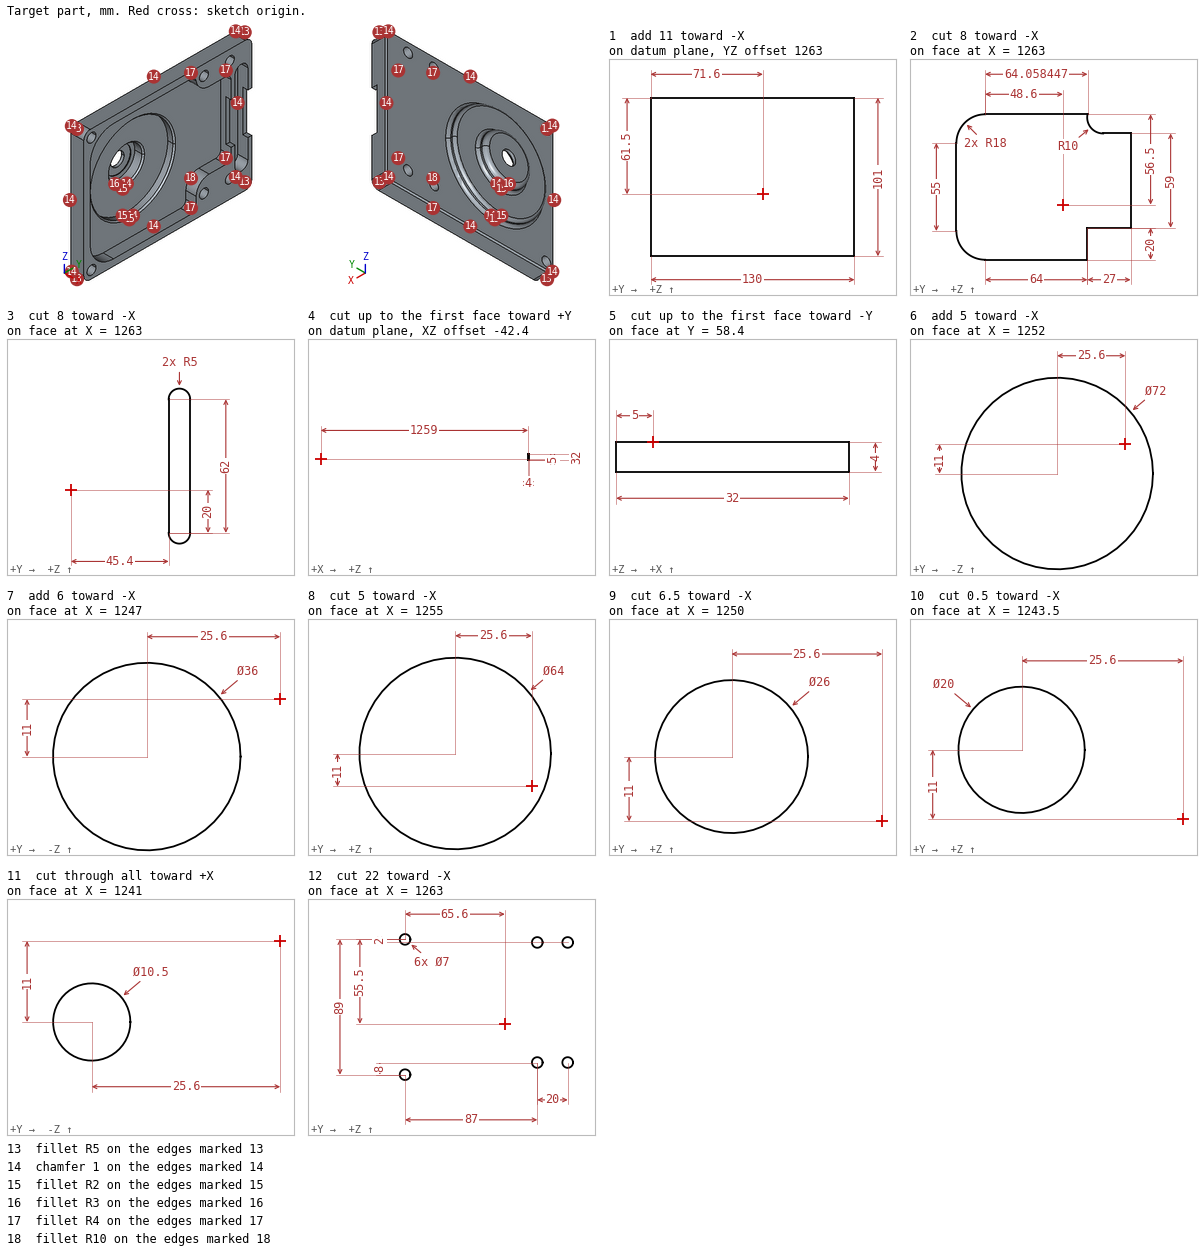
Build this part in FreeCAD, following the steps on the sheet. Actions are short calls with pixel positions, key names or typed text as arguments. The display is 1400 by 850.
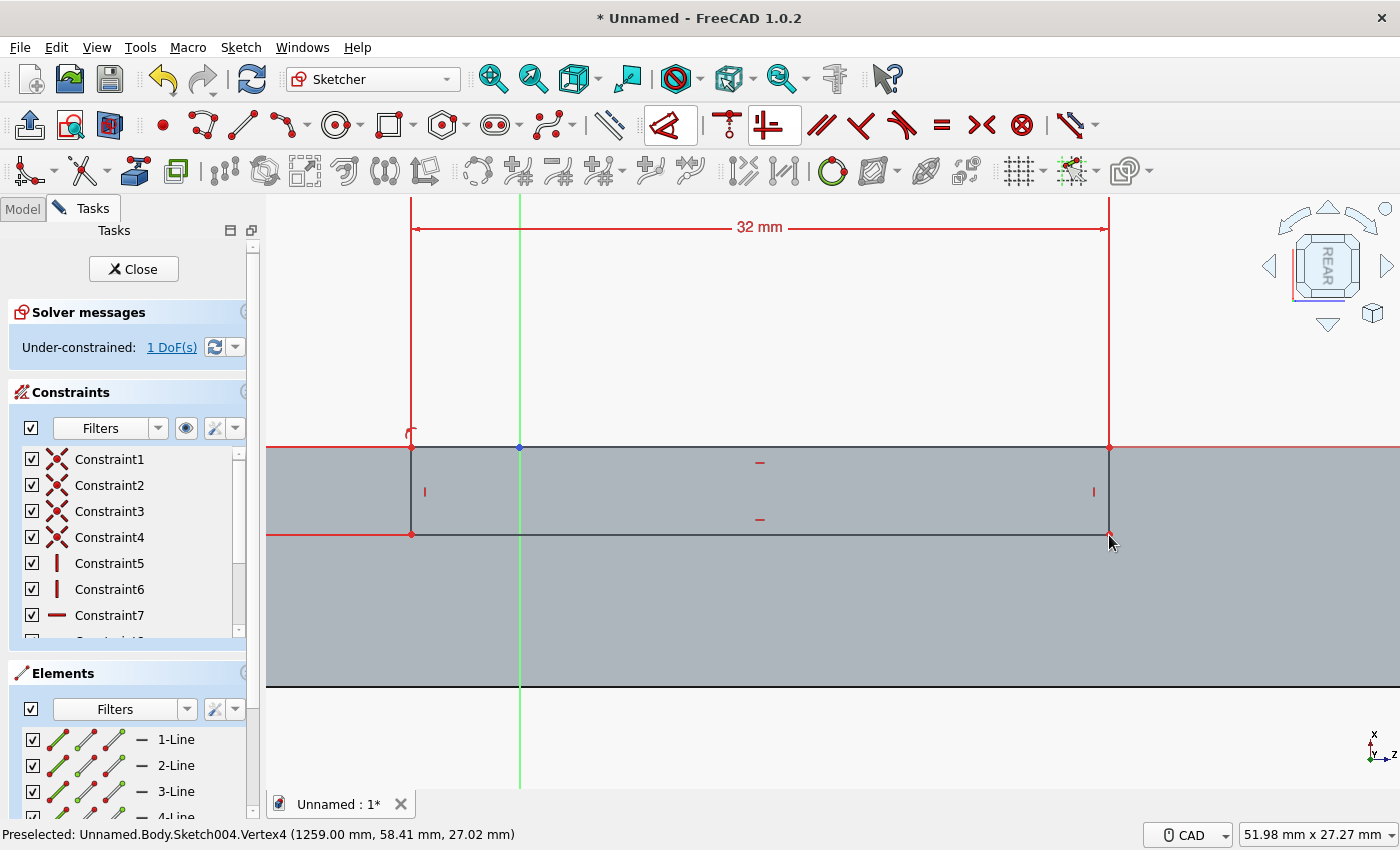
click(411, 447)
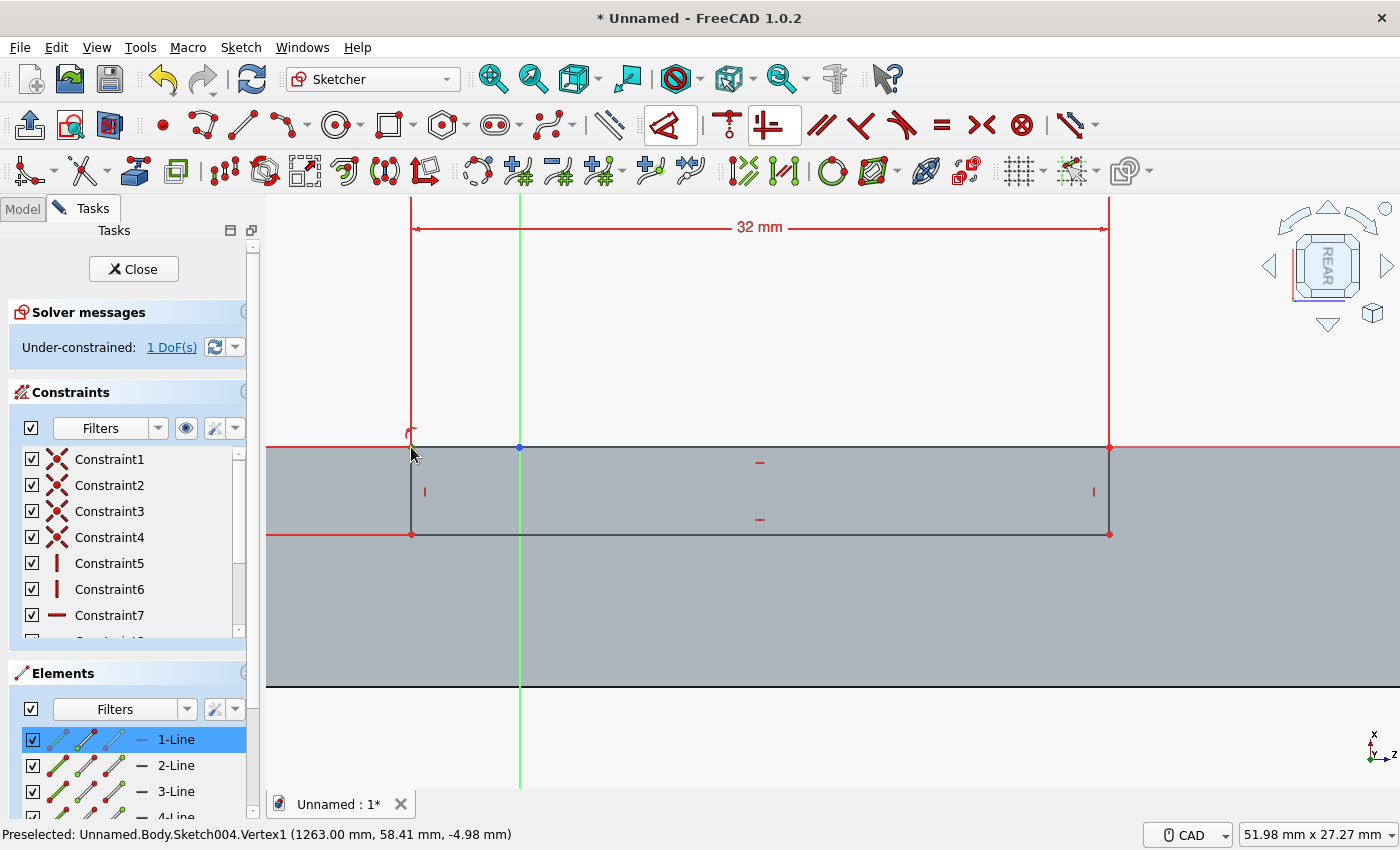
key(l)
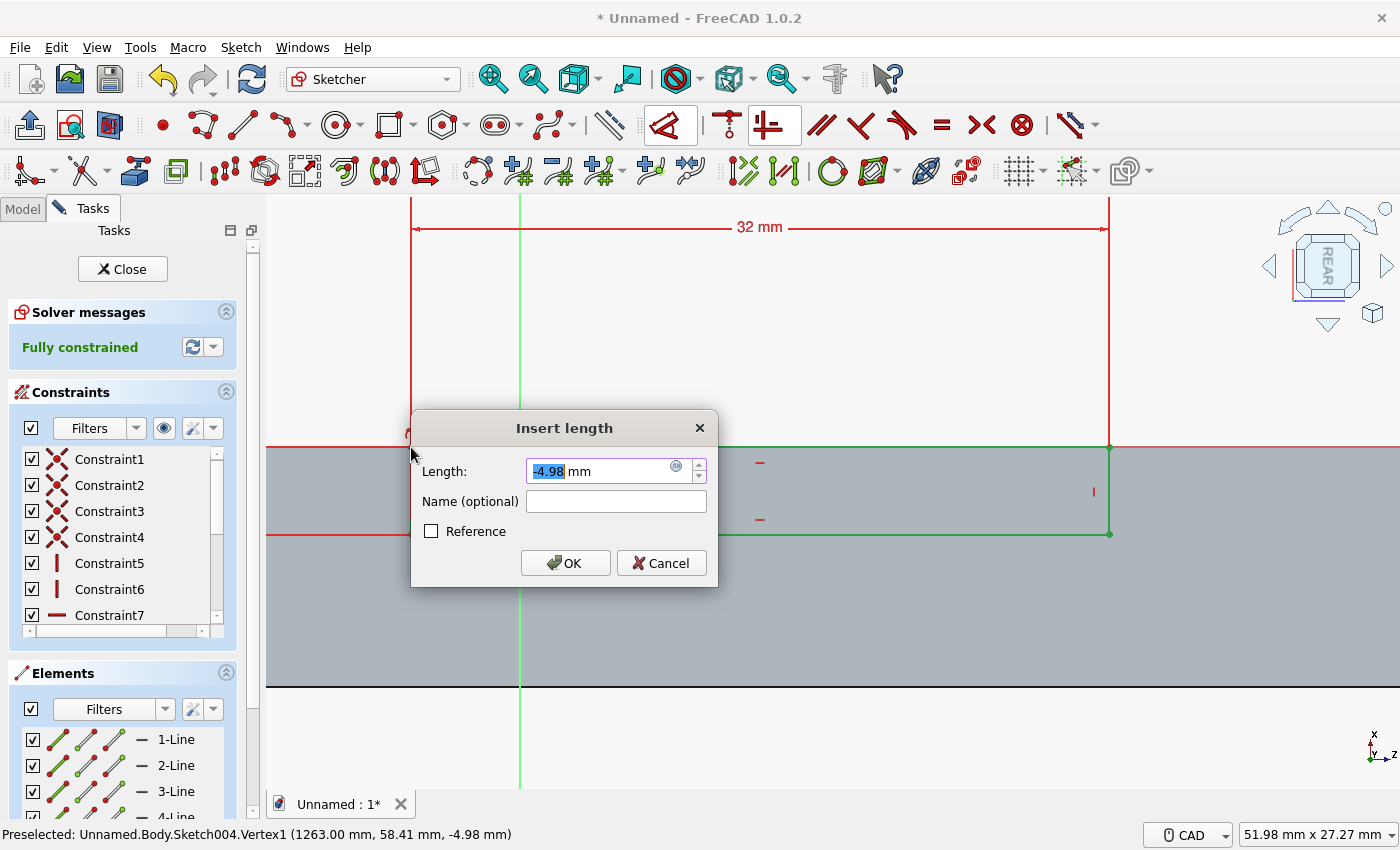
text(-5)
key(Return)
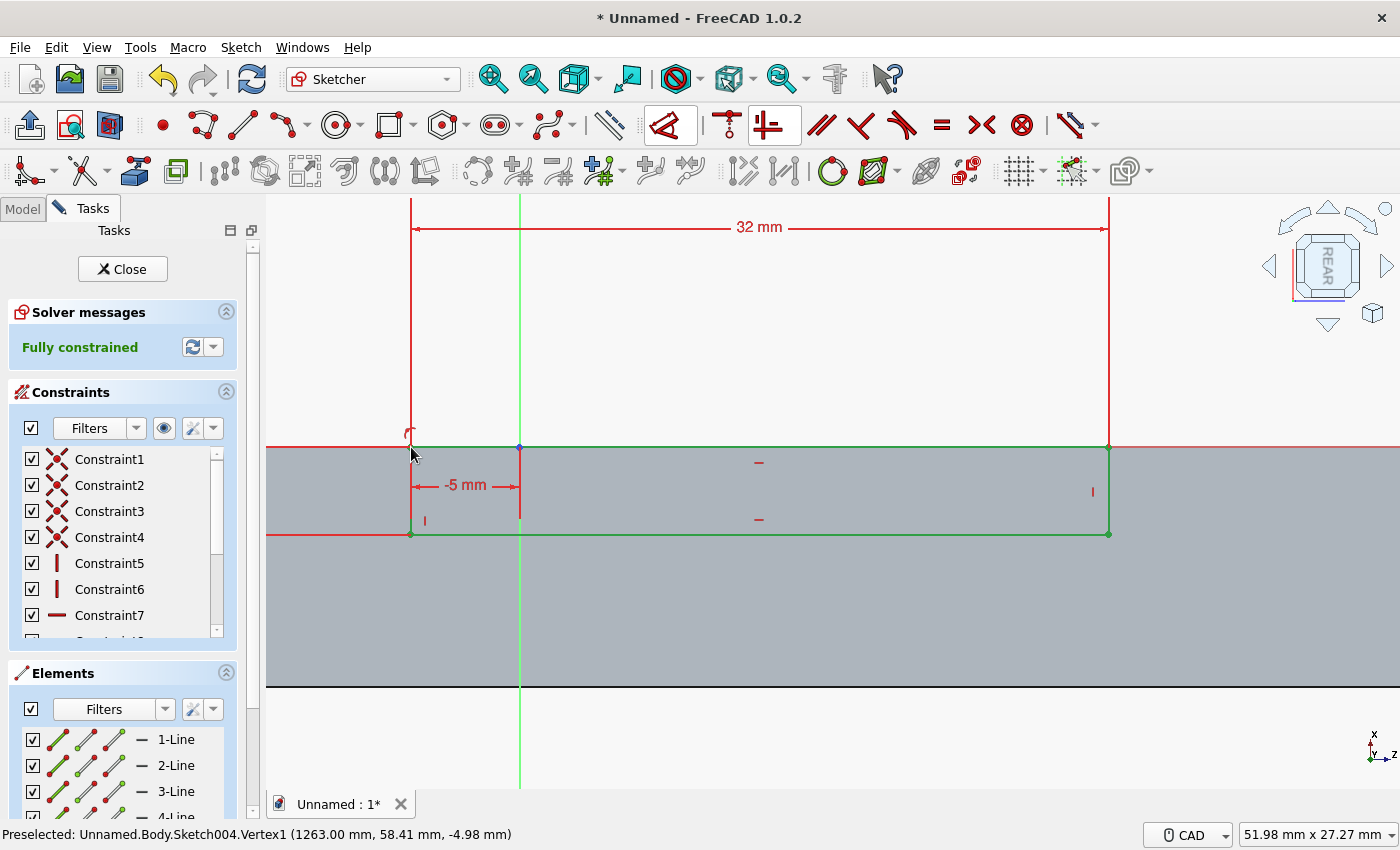
click(123, 269)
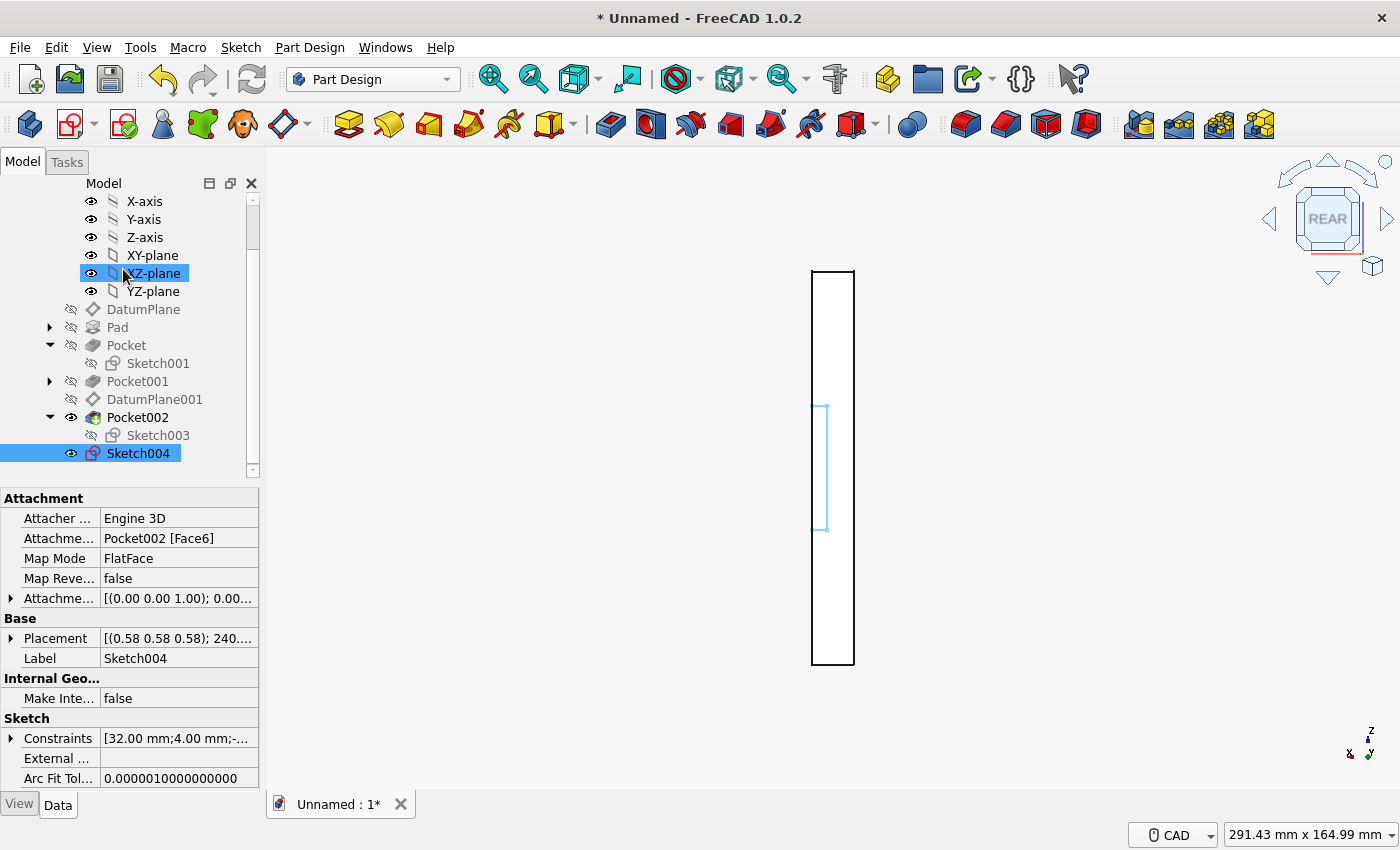
click(612, 124)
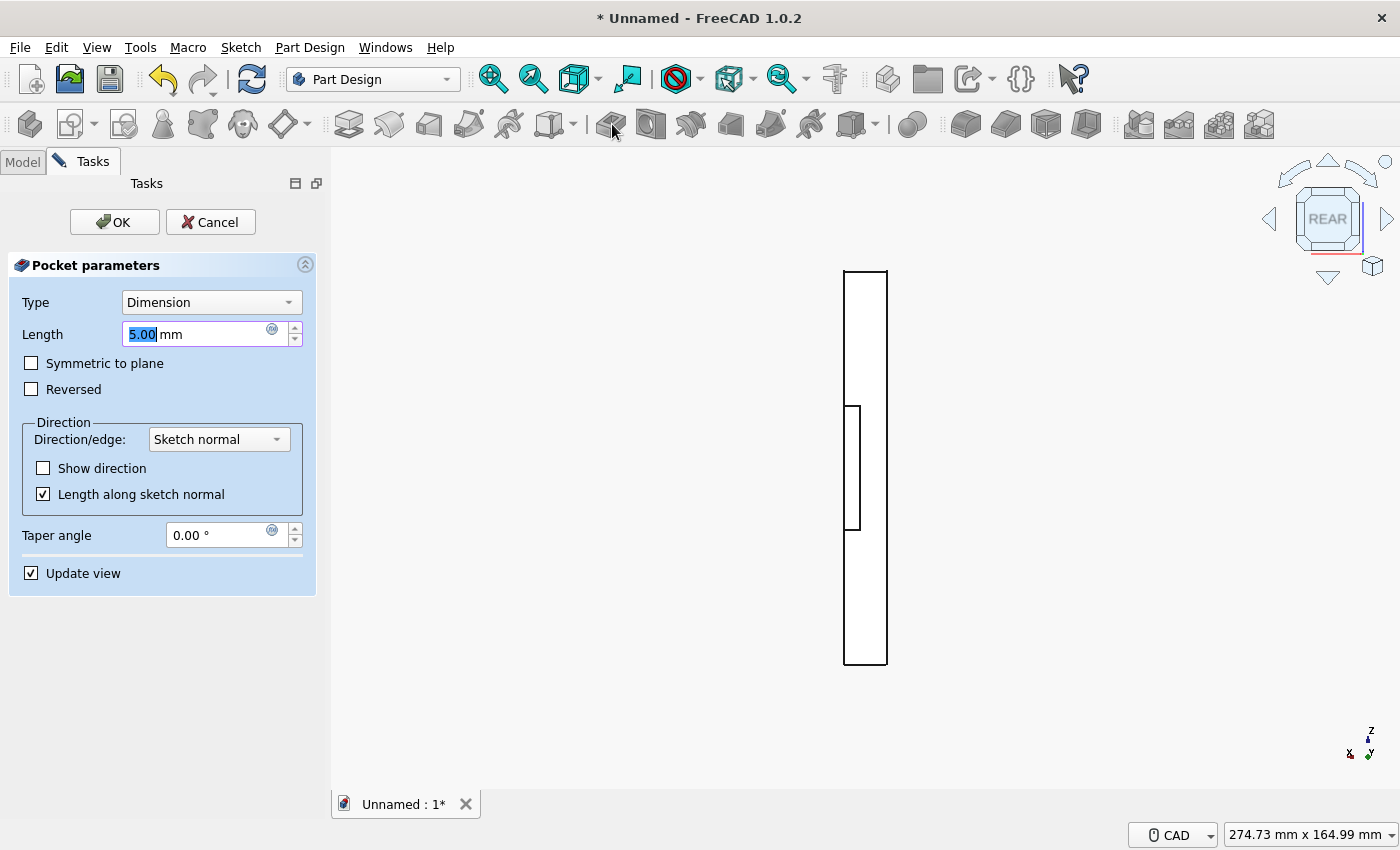
click(212, 302)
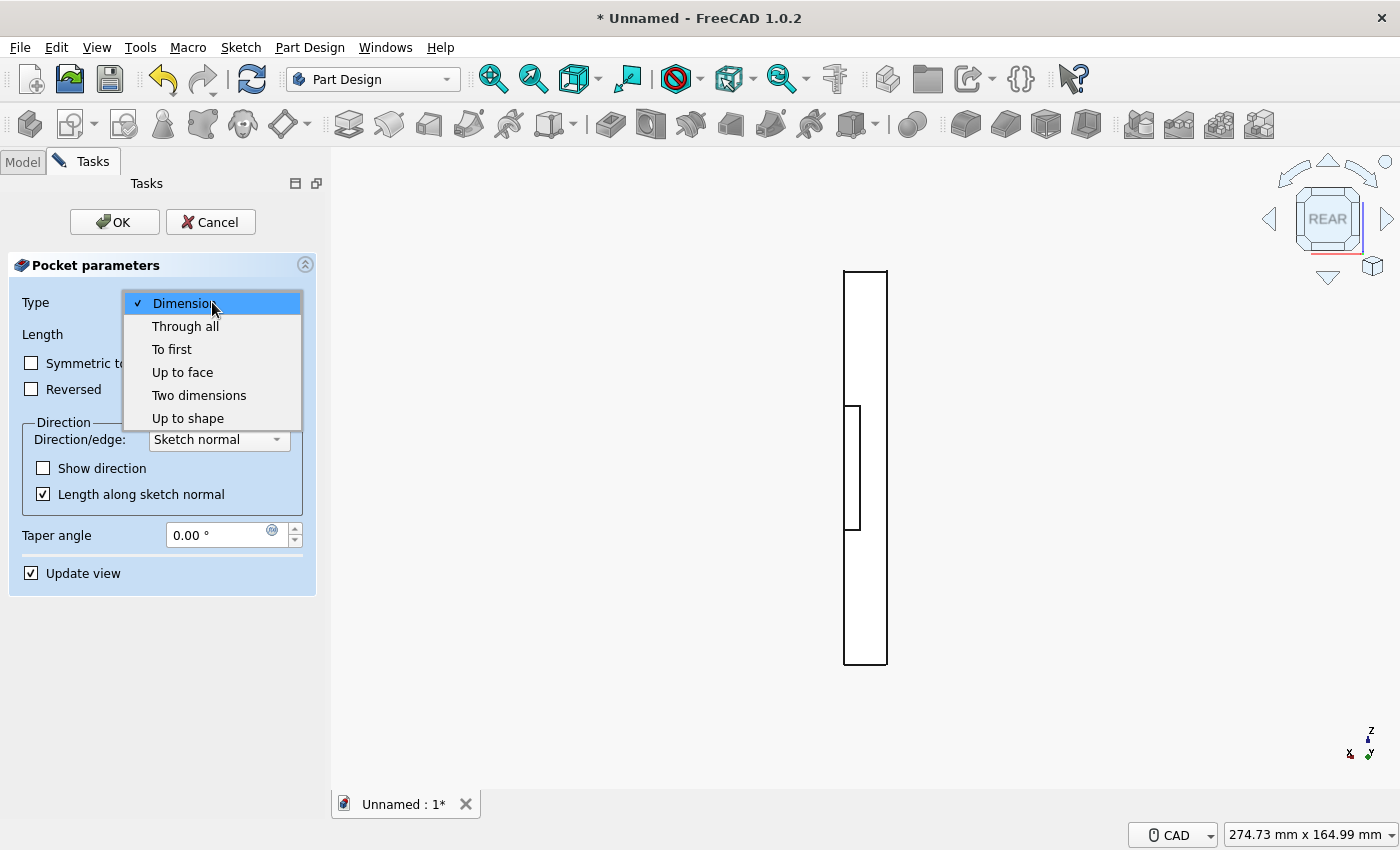
click(212, 350)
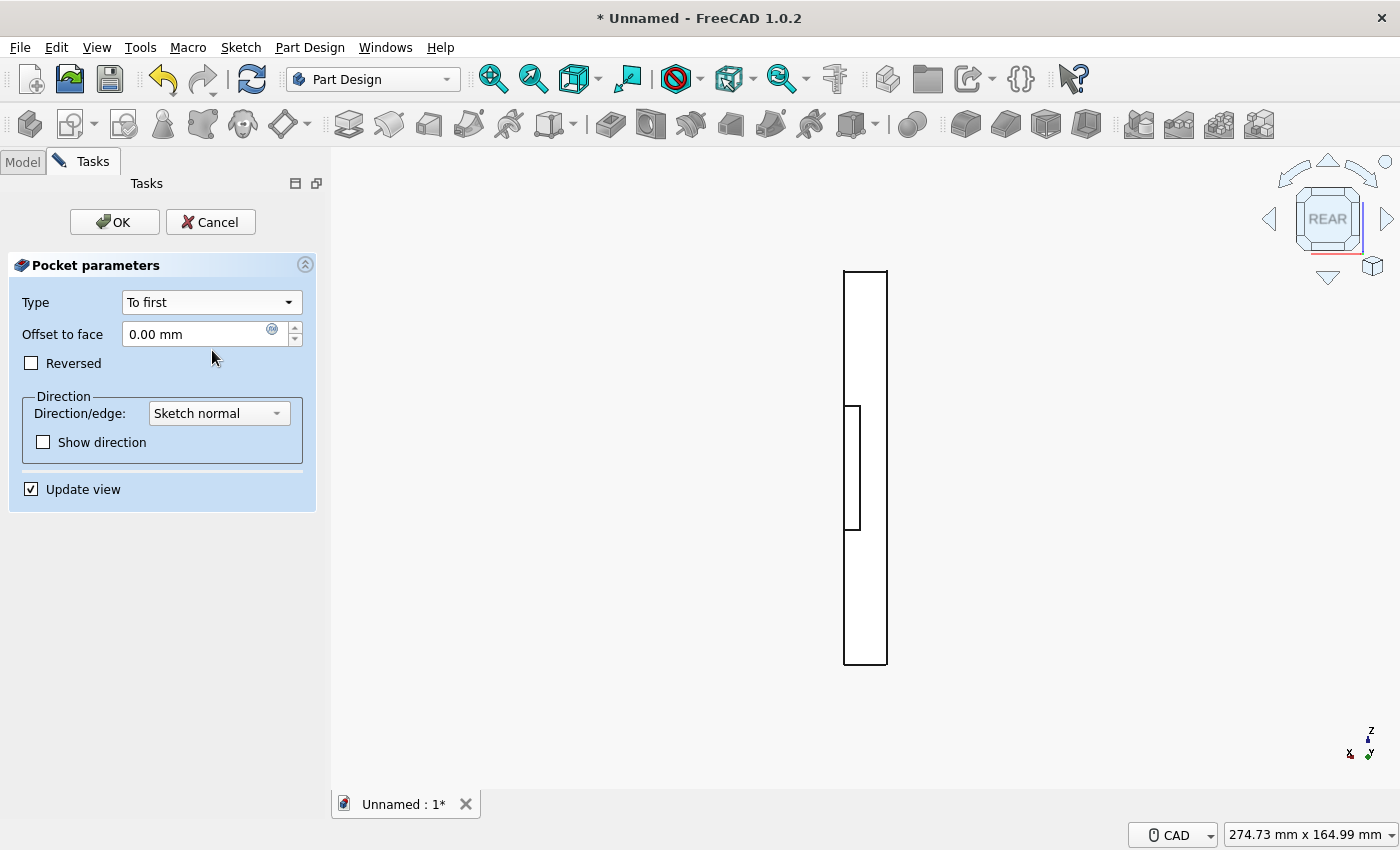
click(115, 222)